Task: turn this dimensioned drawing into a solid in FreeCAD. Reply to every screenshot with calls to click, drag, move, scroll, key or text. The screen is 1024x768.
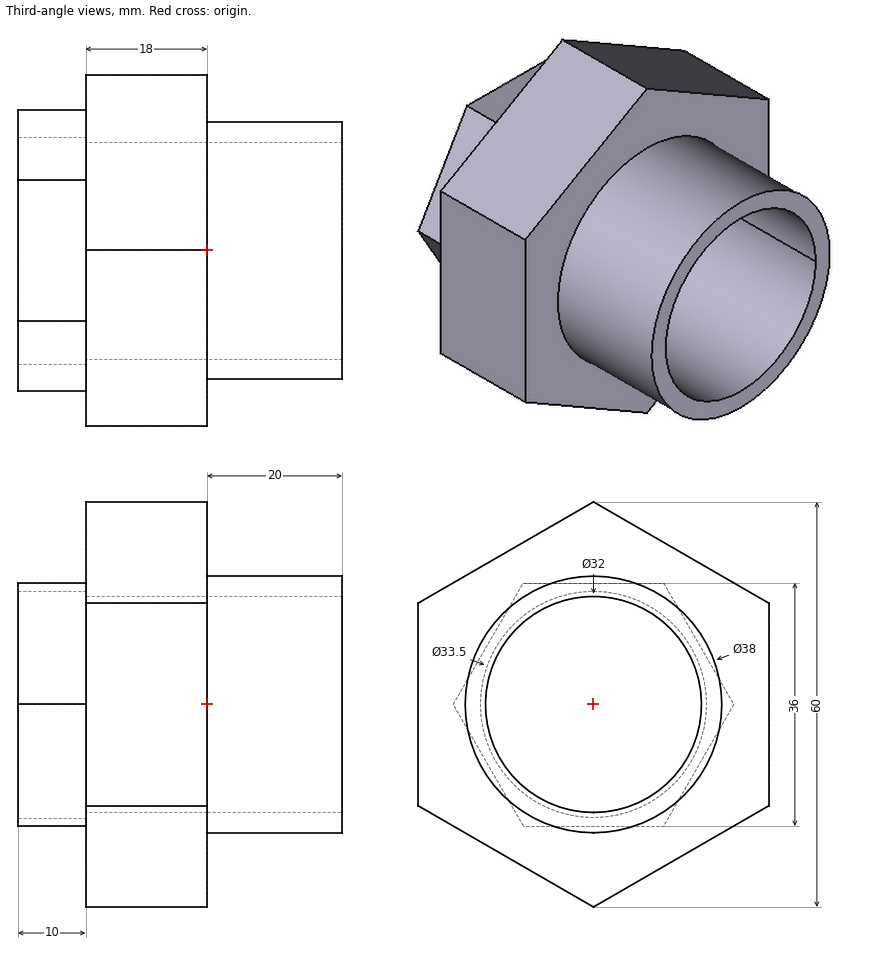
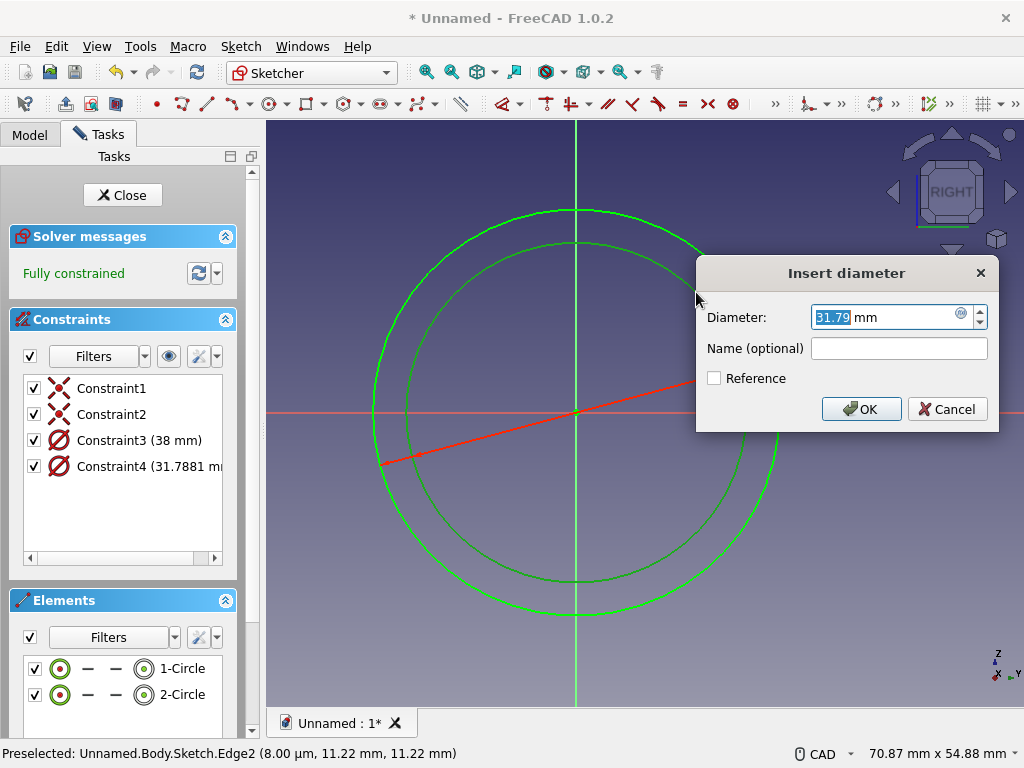
text(32)
key(Return)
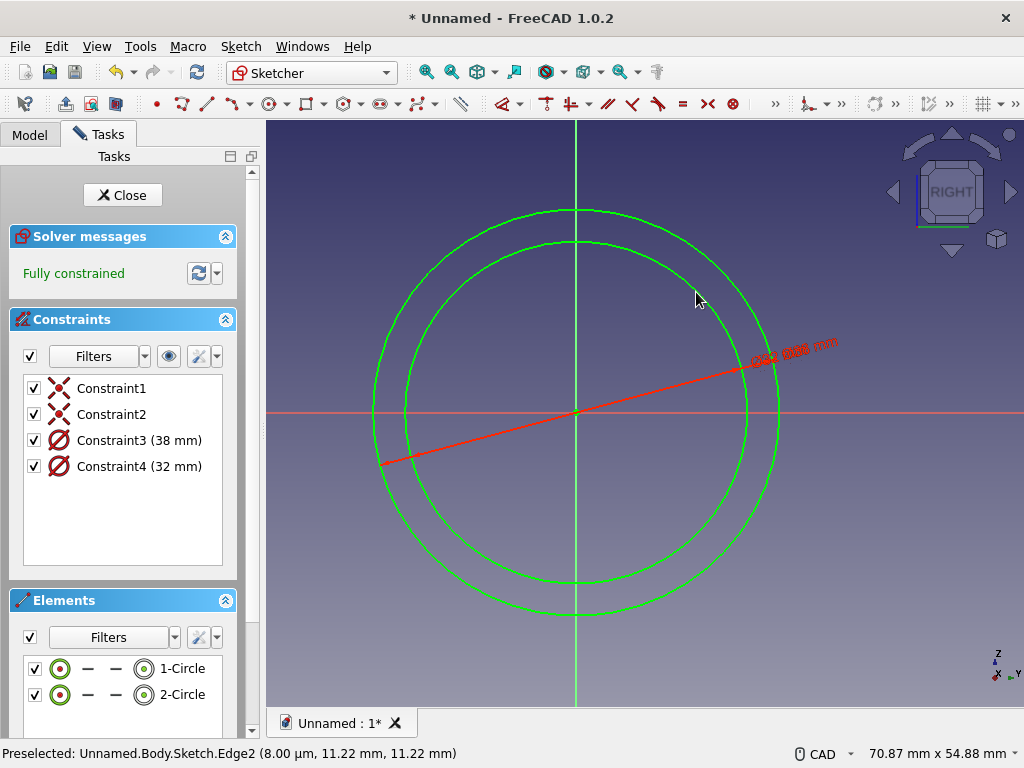
click(123, 195)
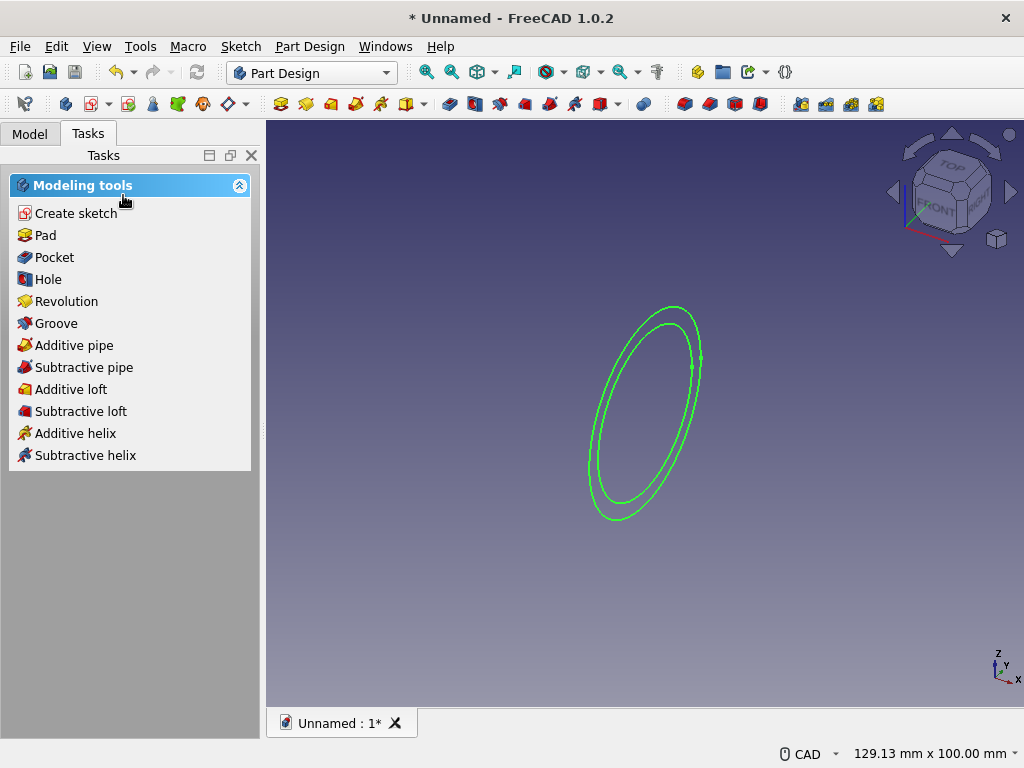
click(281, 104)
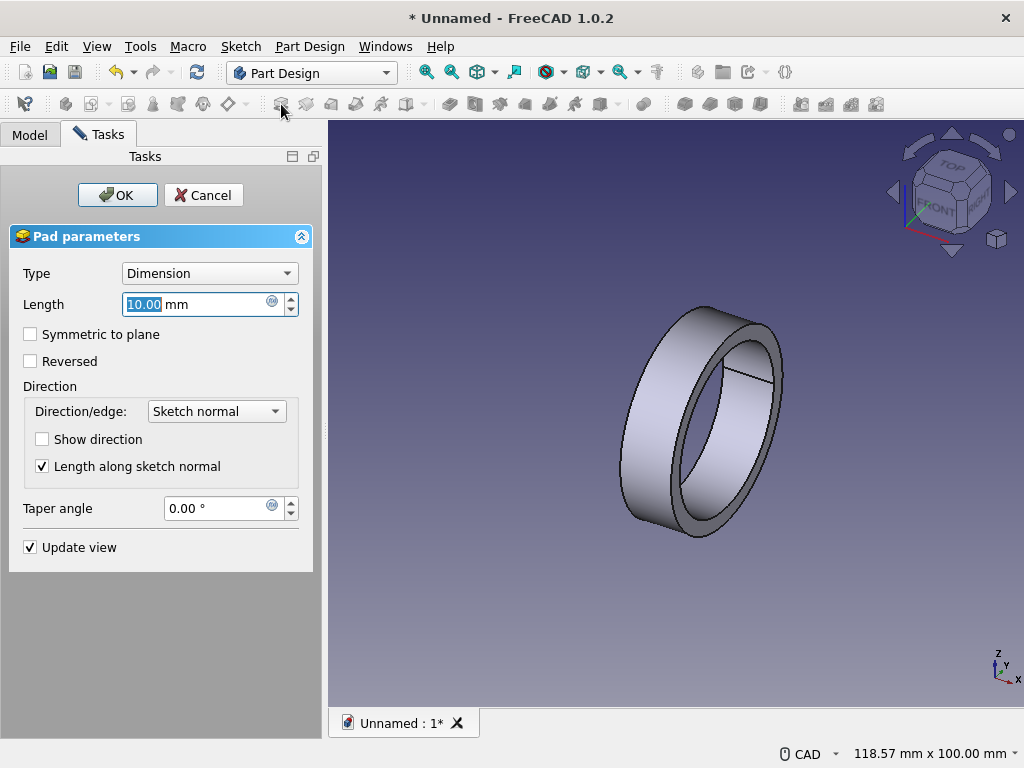
text(20)
key(Tab)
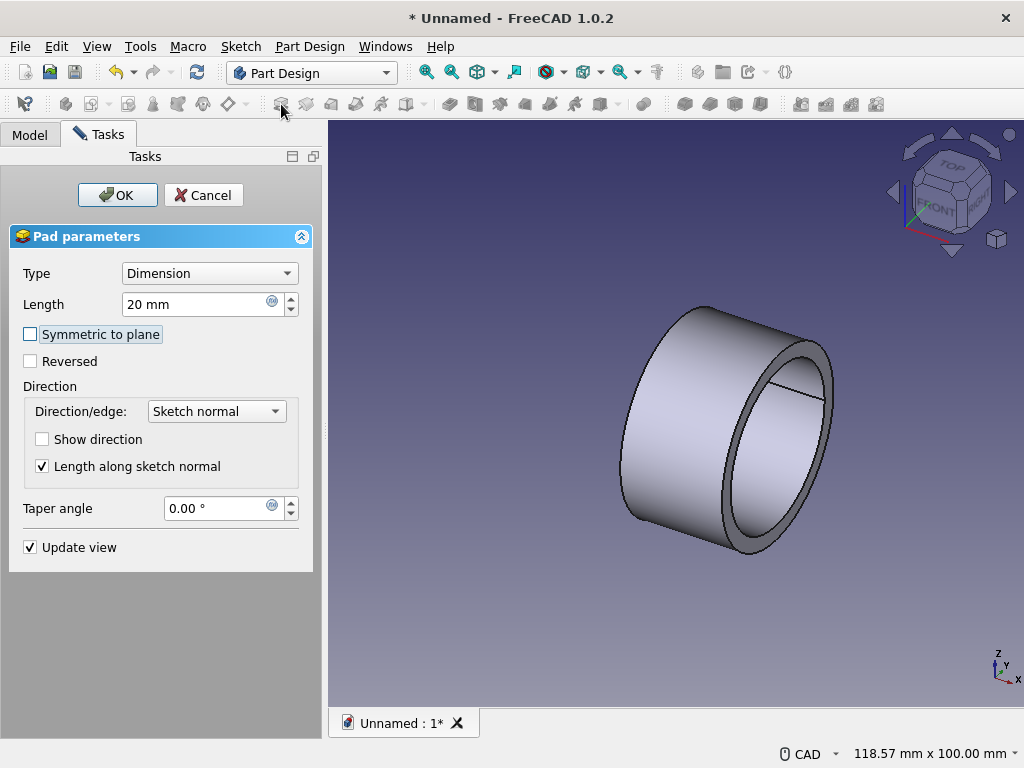
click(118, 195)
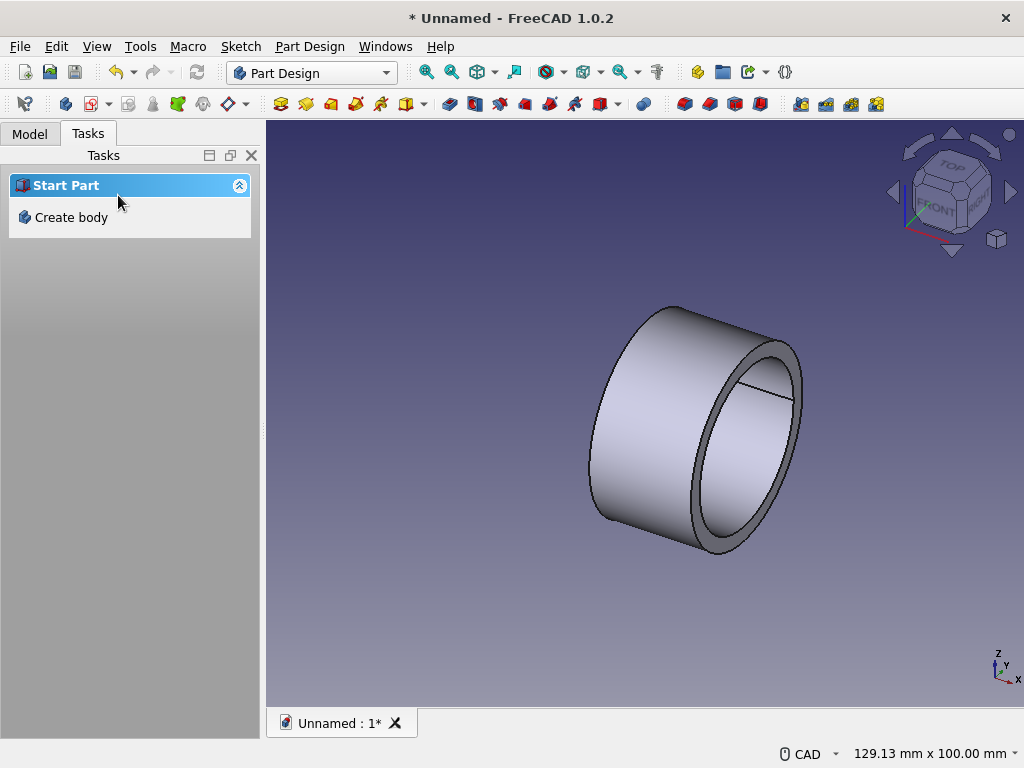
click(30, 134)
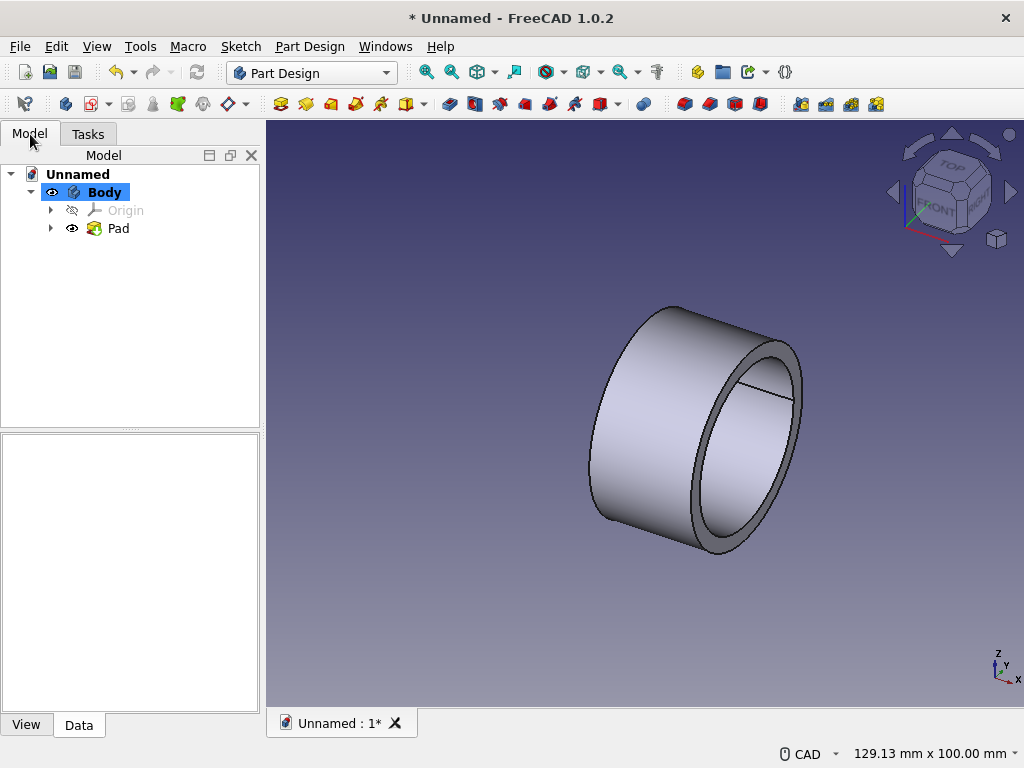
click(51, 210)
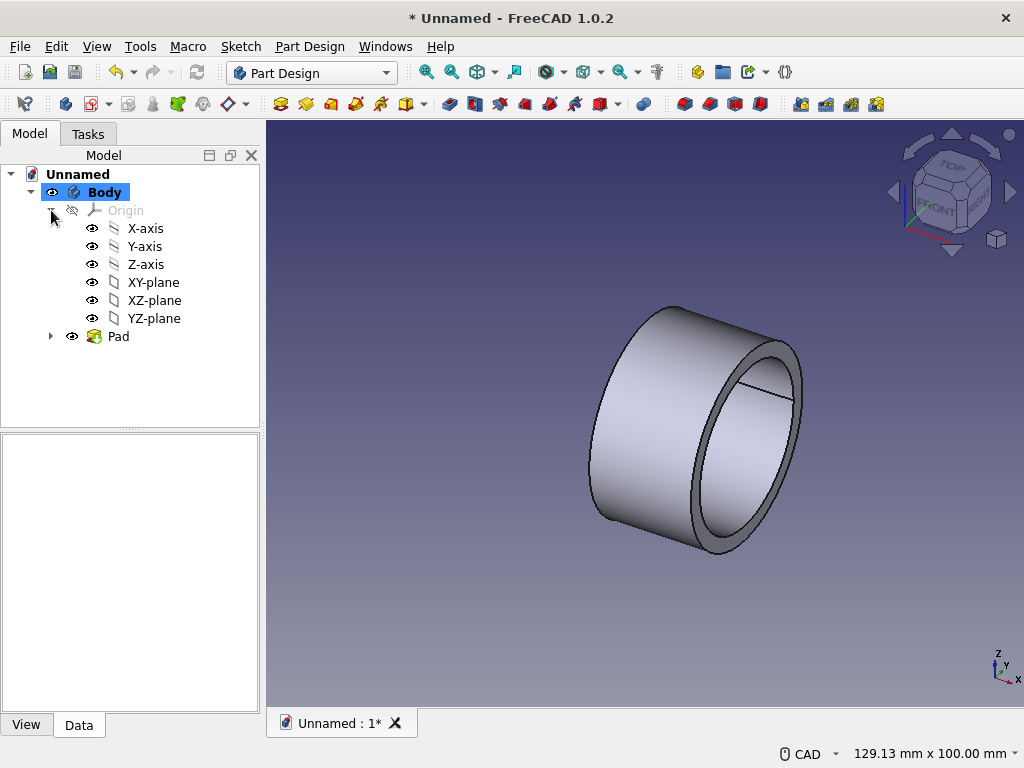
click(137, 318)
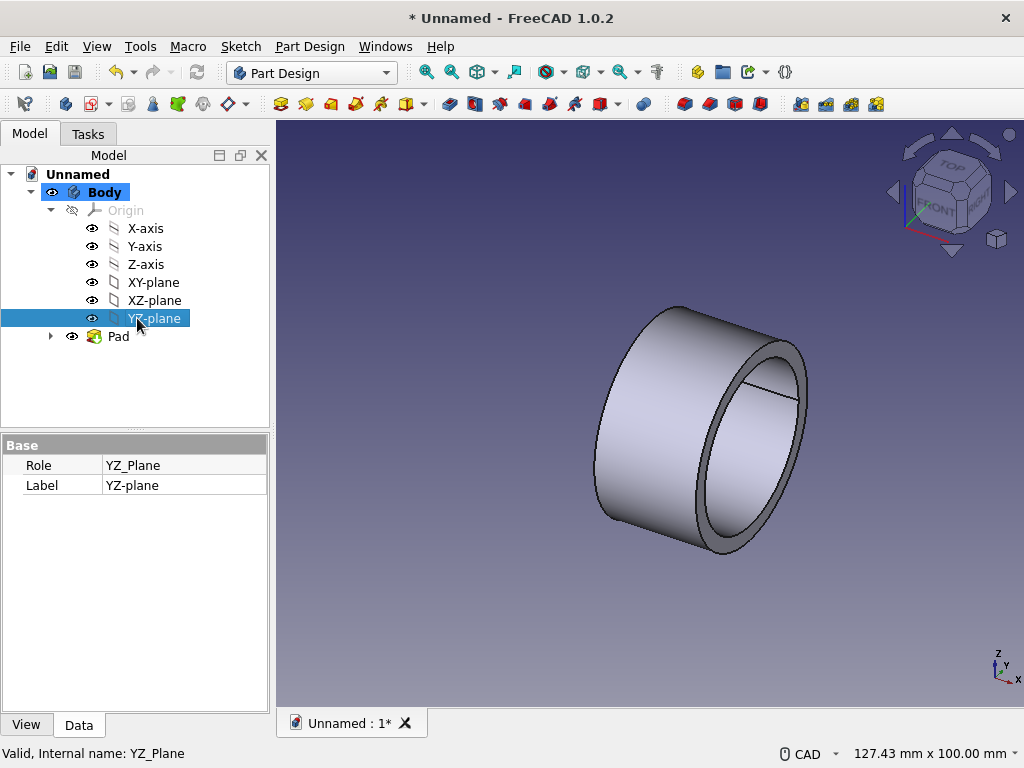
click(228, 104)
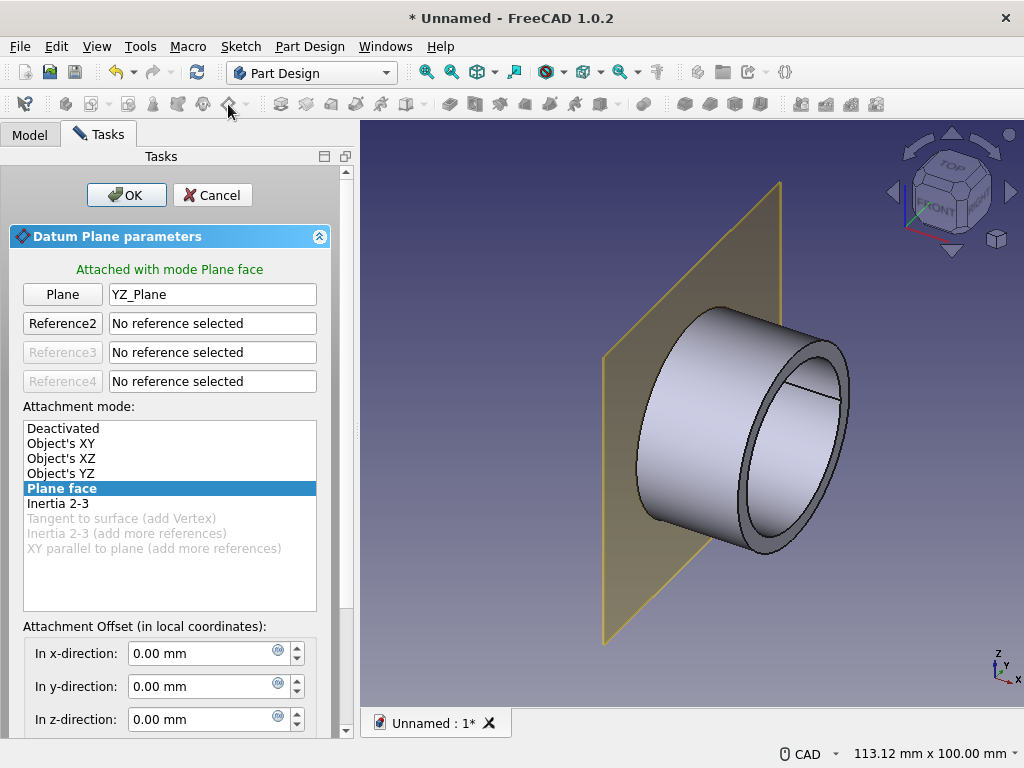
triple_click(210, 720)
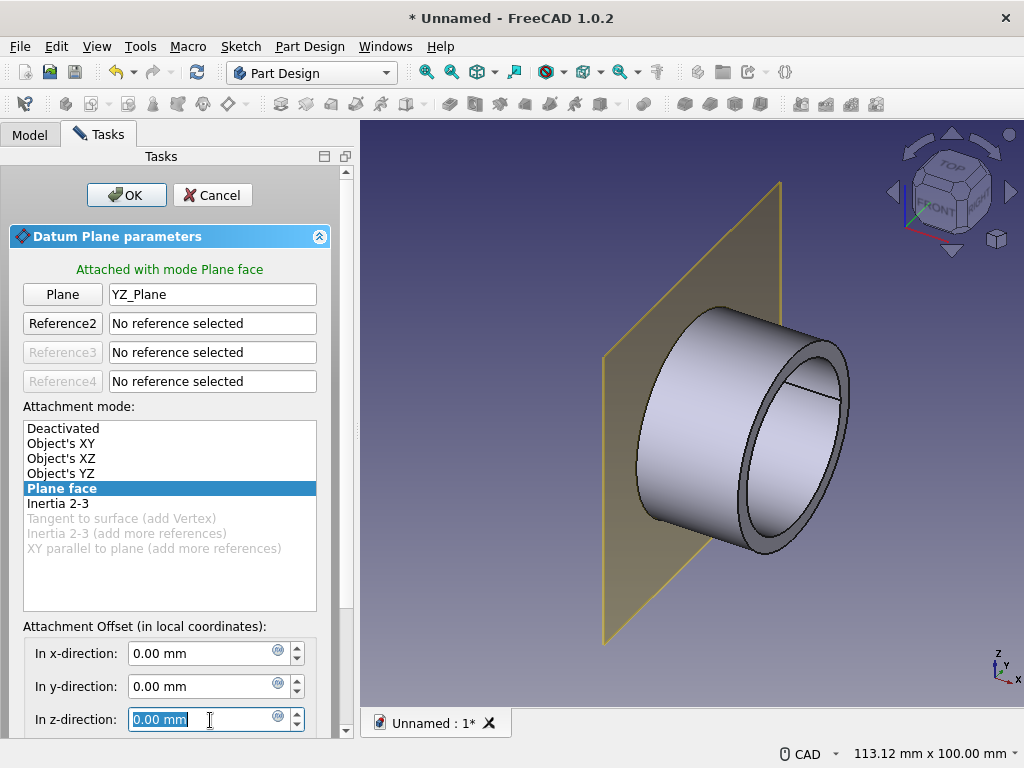
text(-18)
key(Tab)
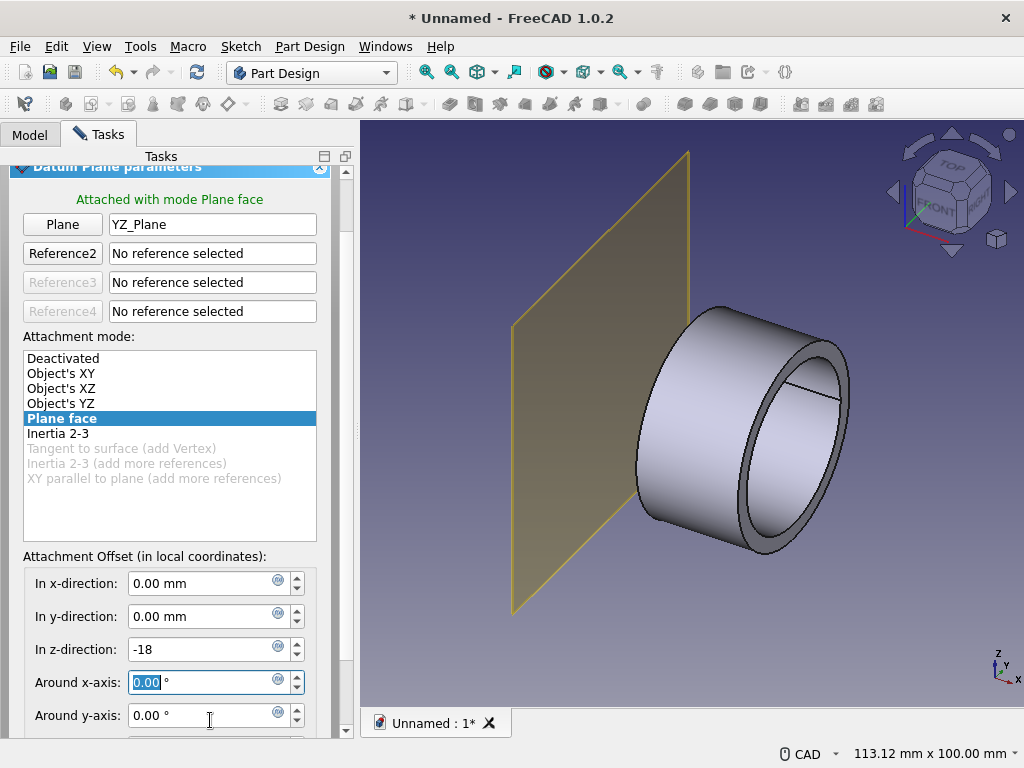
scroll(346, 452, up, 2)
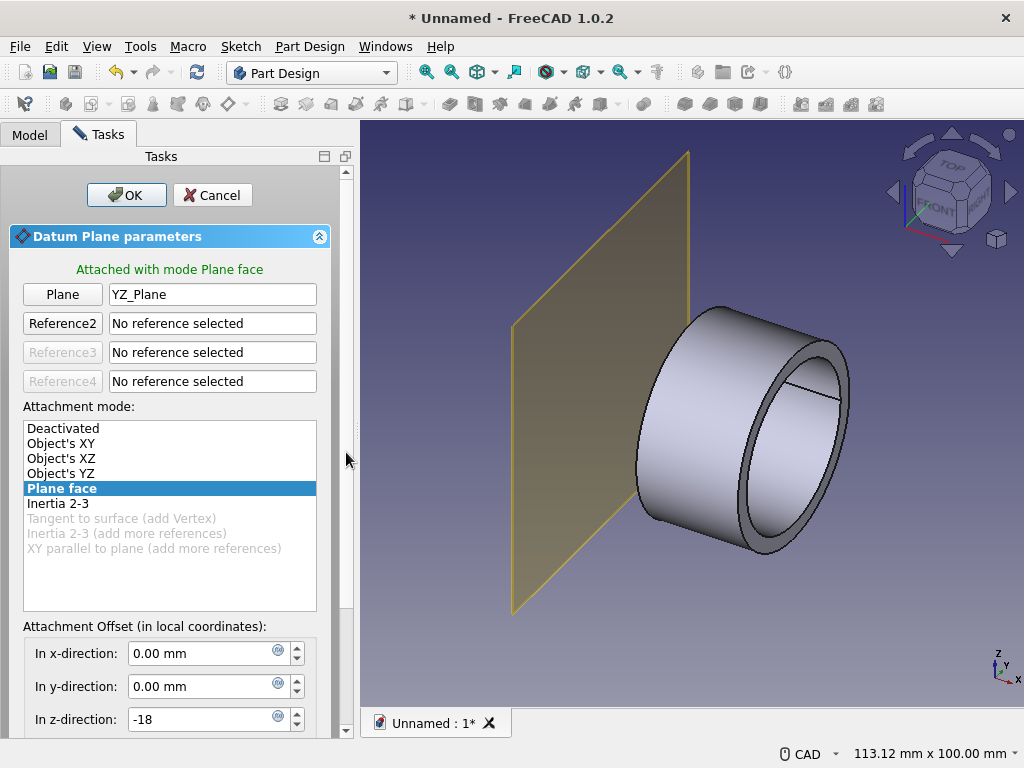
click(127, 195)